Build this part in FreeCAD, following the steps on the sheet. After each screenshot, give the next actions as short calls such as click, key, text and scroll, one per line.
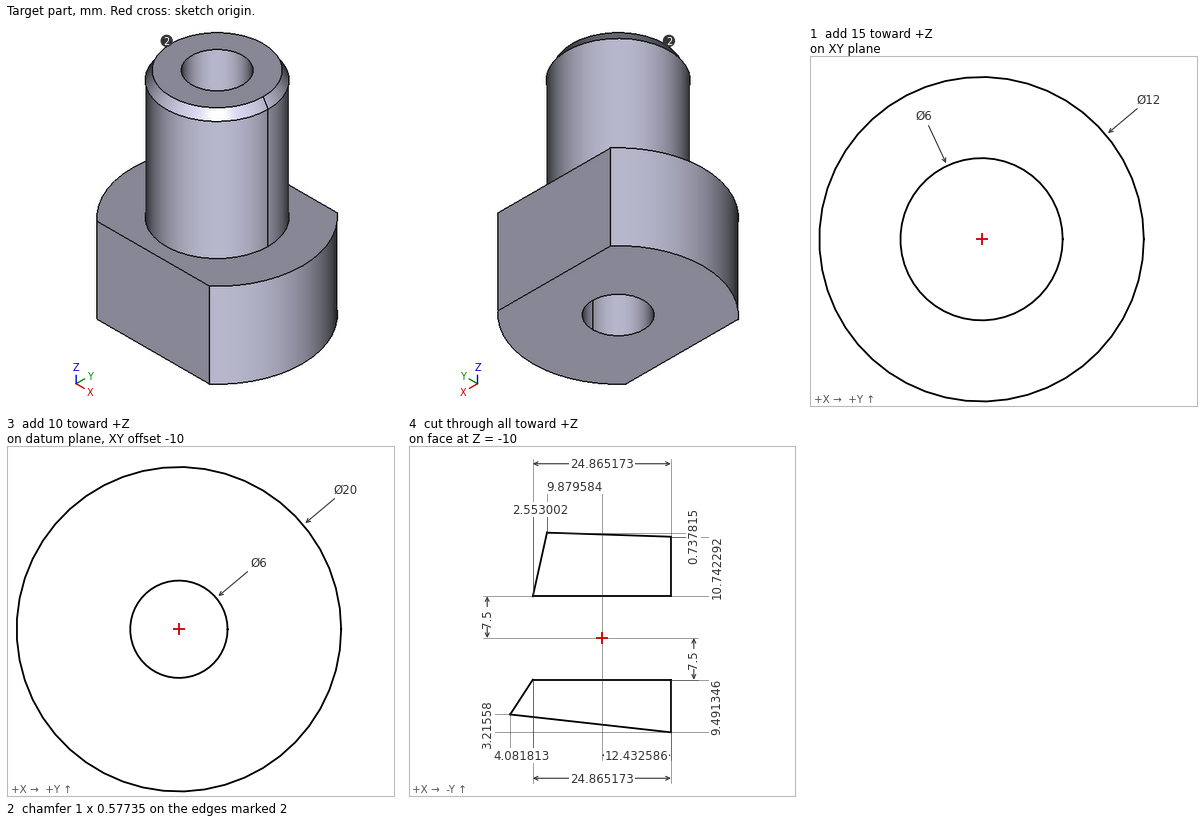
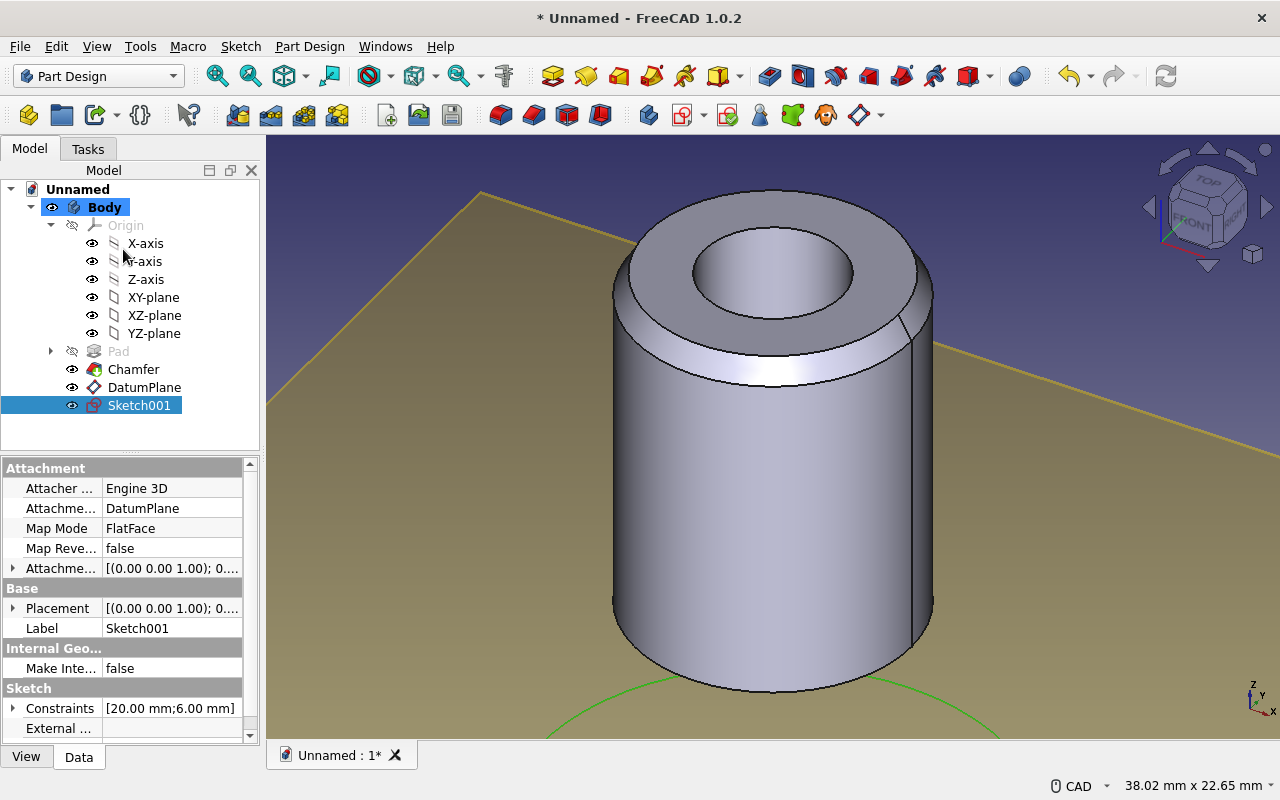
click(553, 76)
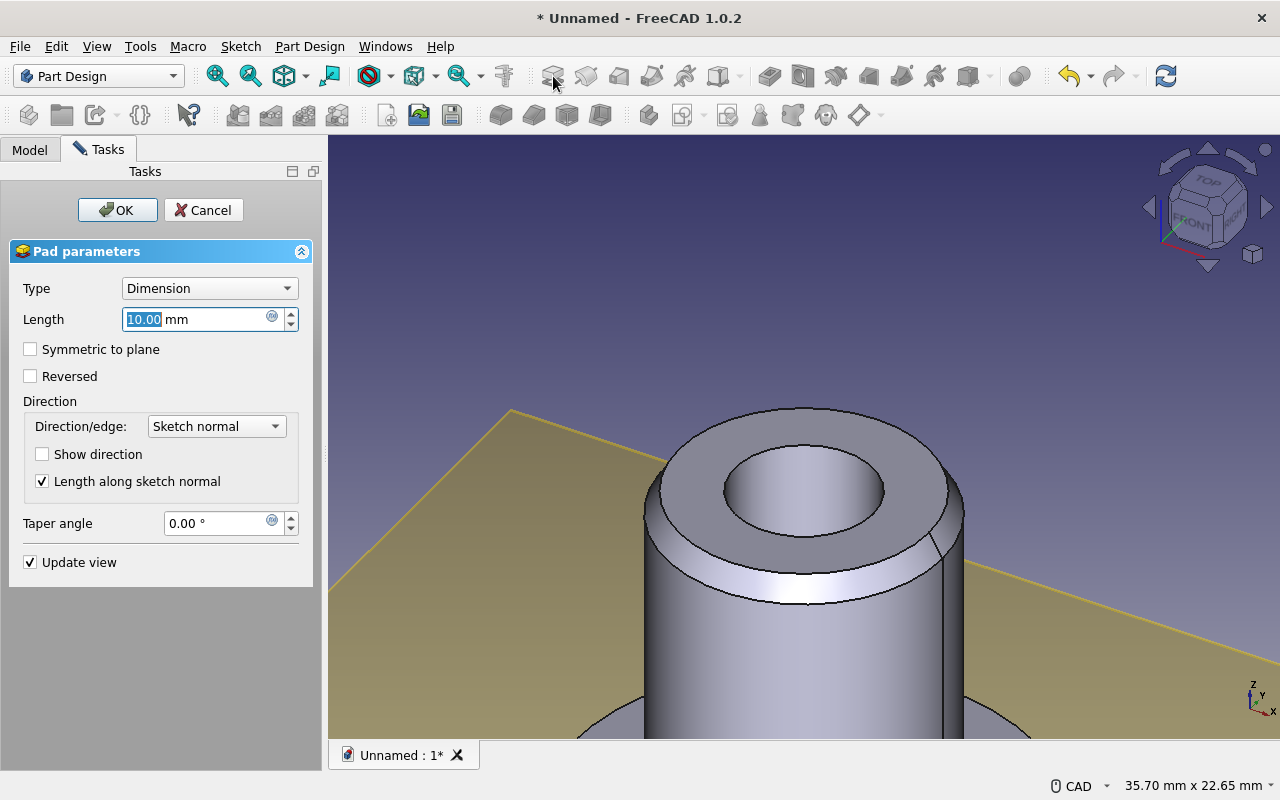
text(10)
key(Tab)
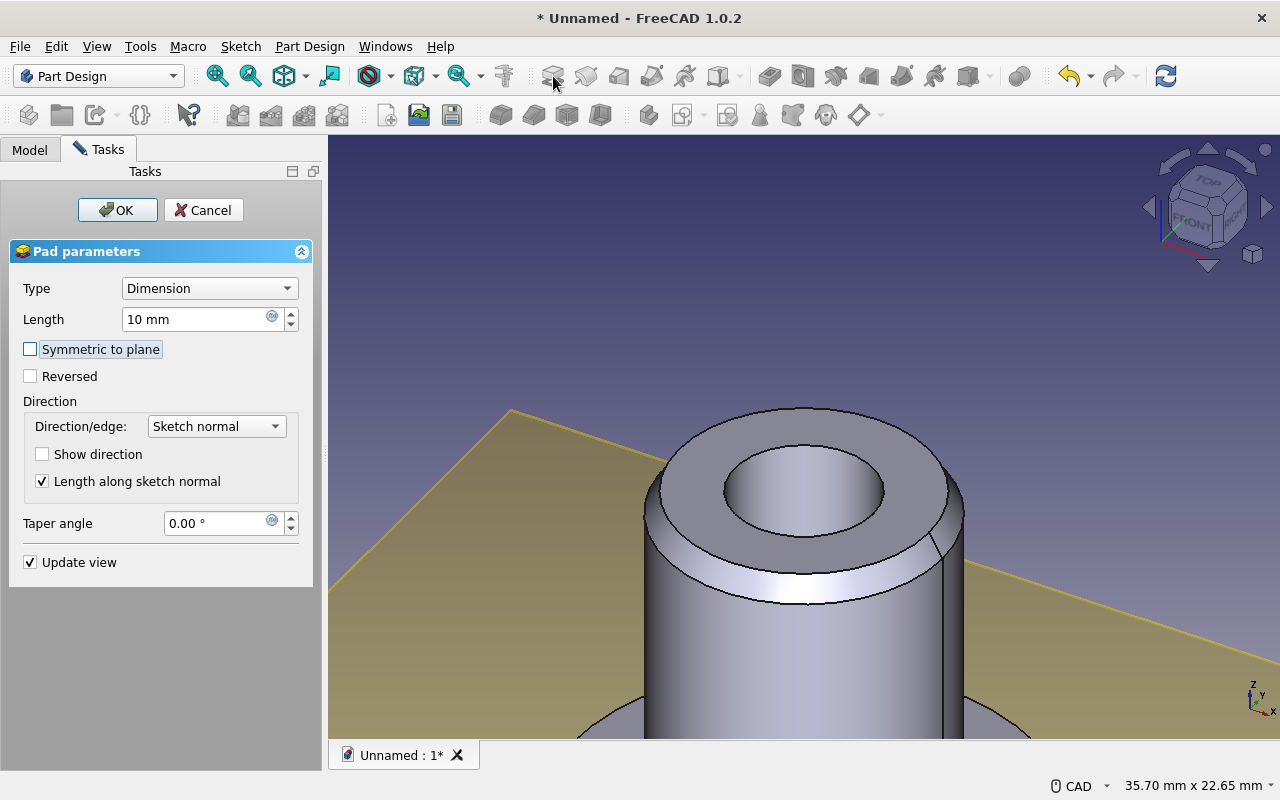
click(118, 210)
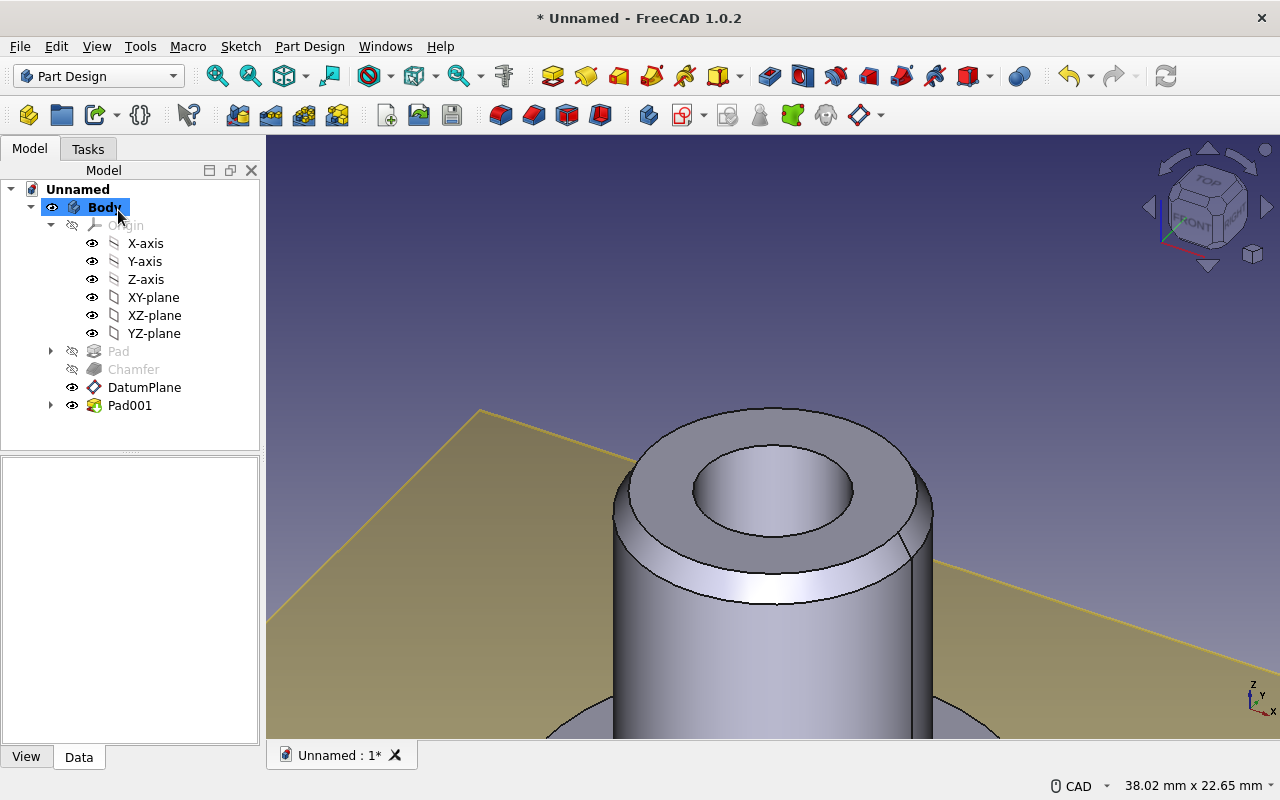
click(117, 387)
key(space)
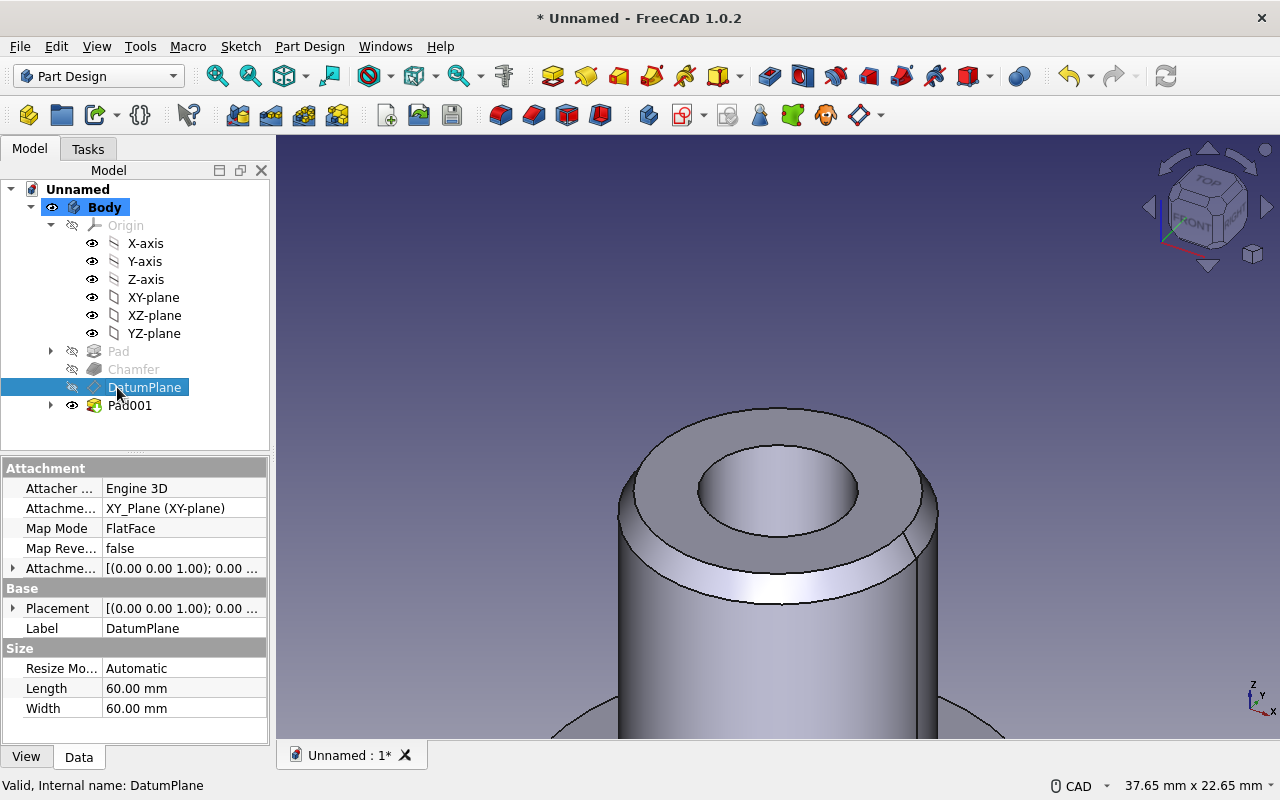
key(v)
key(f)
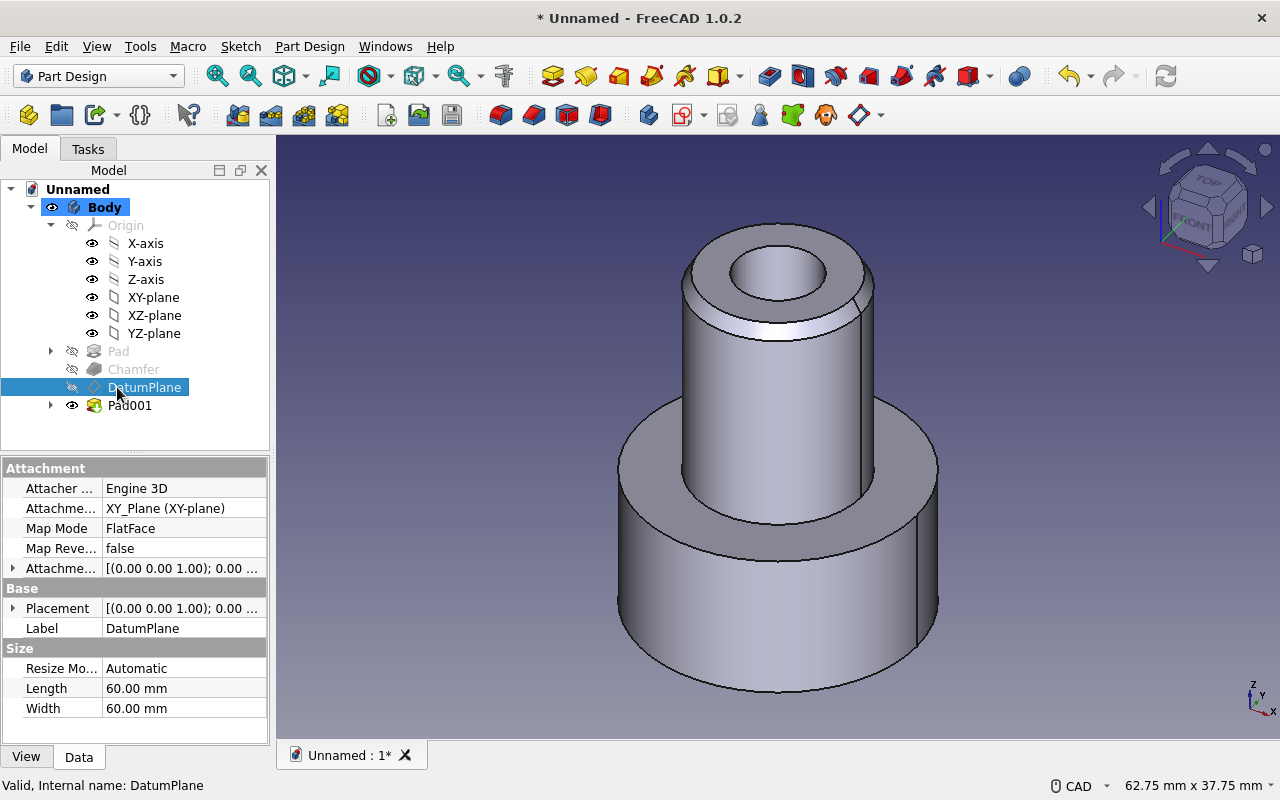
key(5)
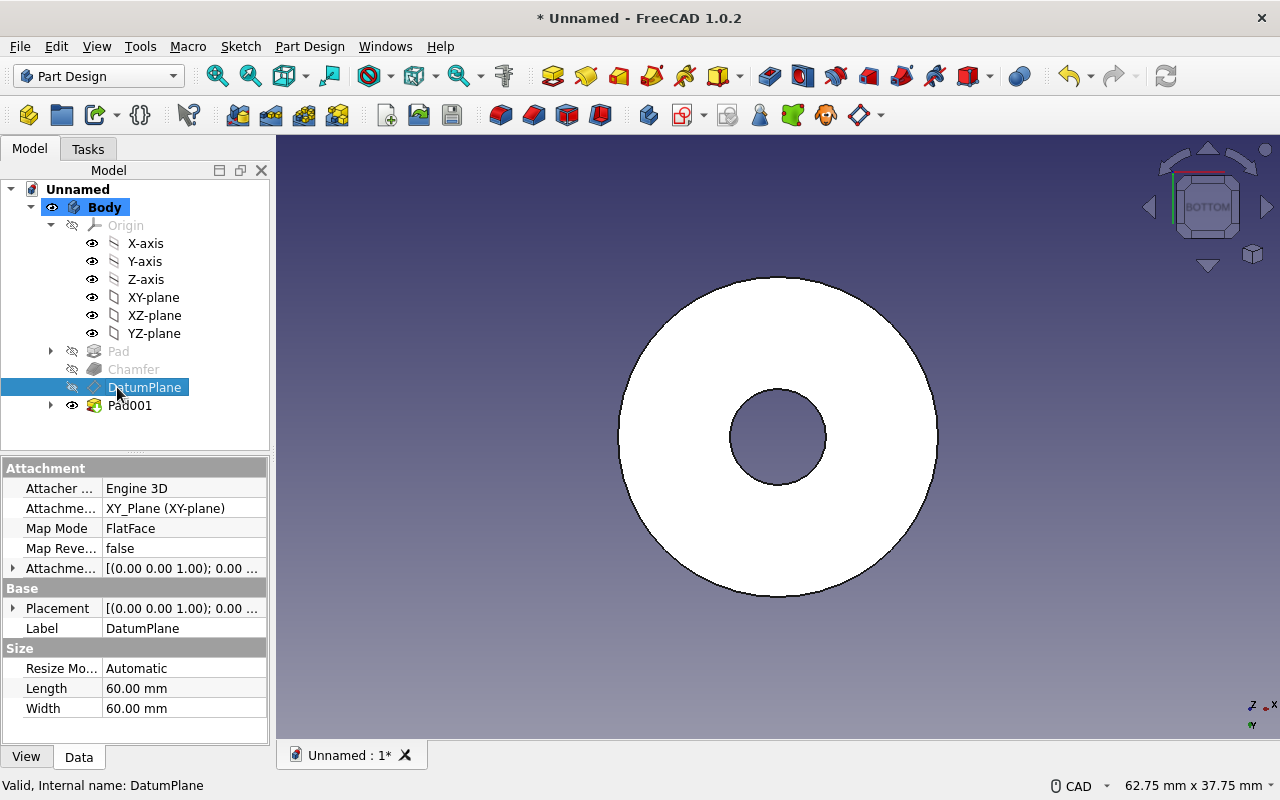
click(687, 482)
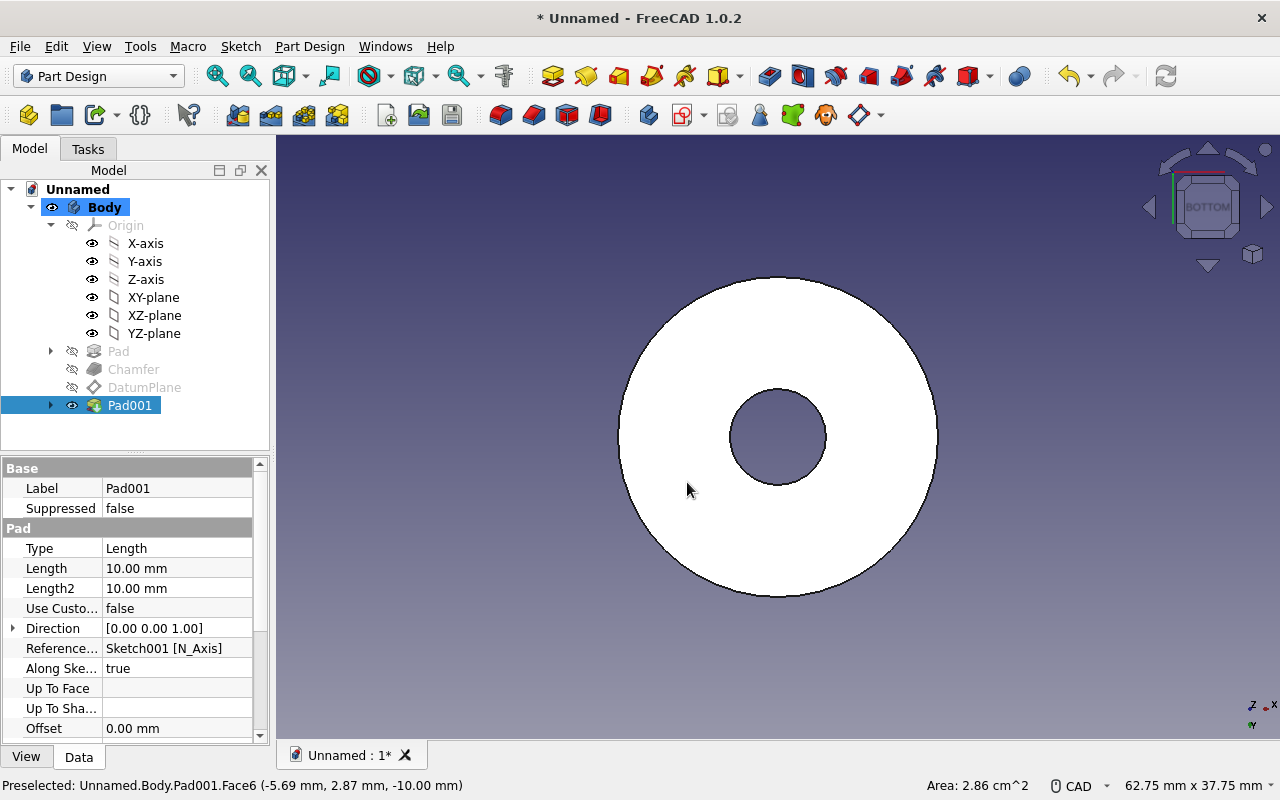
click(682, 116)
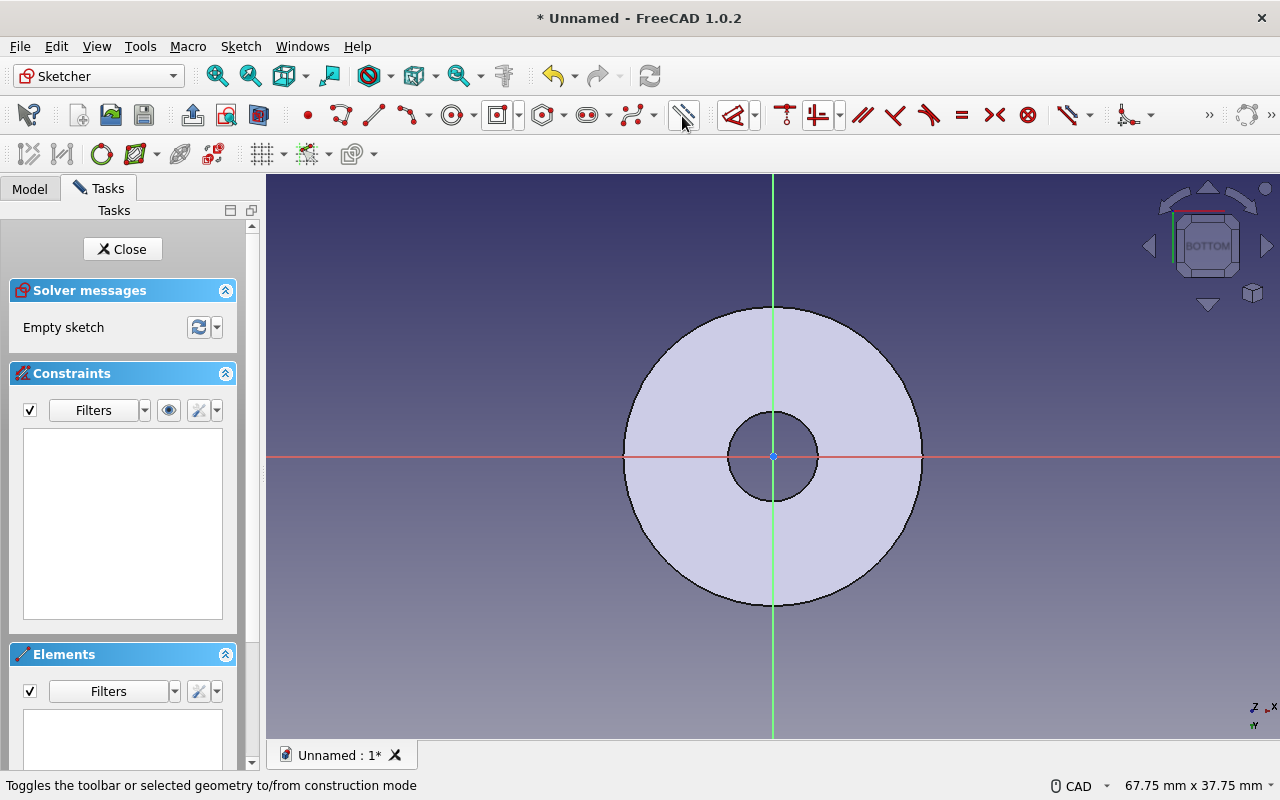
scroll(627, 487, down, 2)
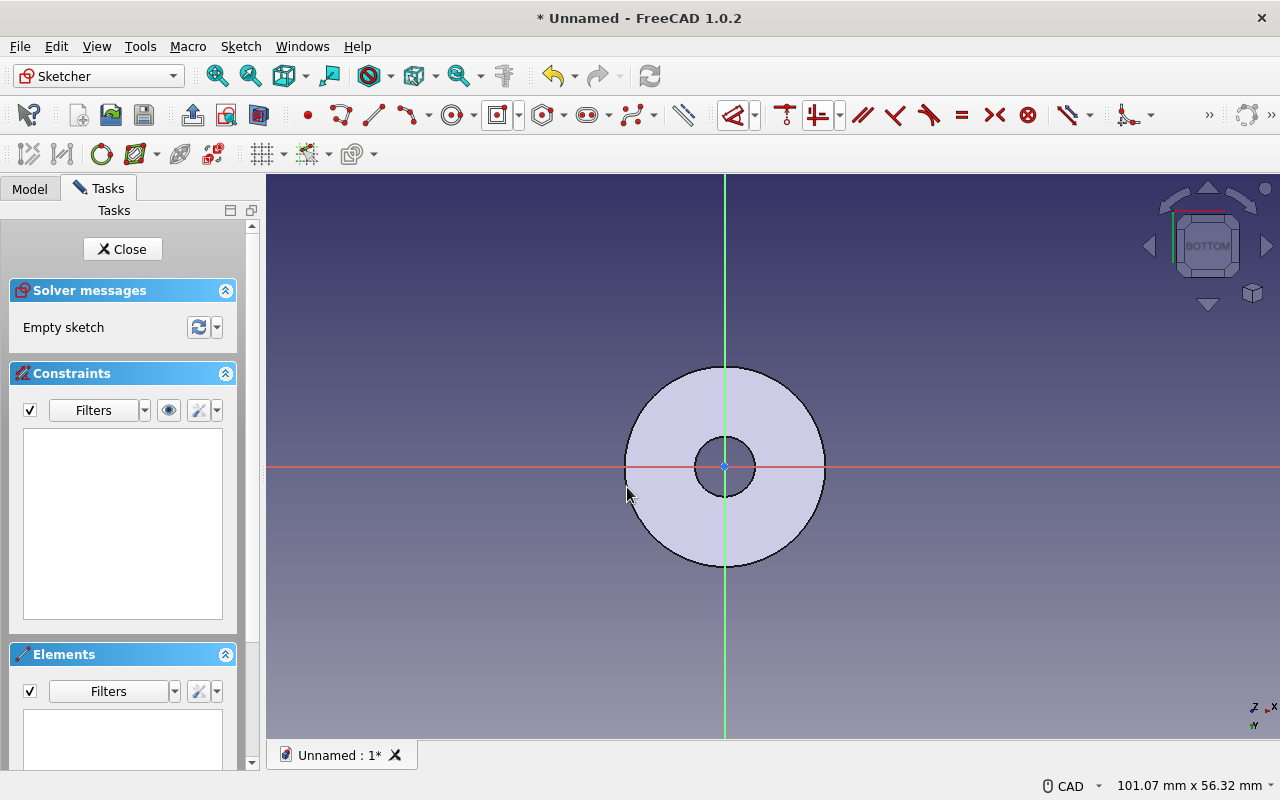
click(341, 116)